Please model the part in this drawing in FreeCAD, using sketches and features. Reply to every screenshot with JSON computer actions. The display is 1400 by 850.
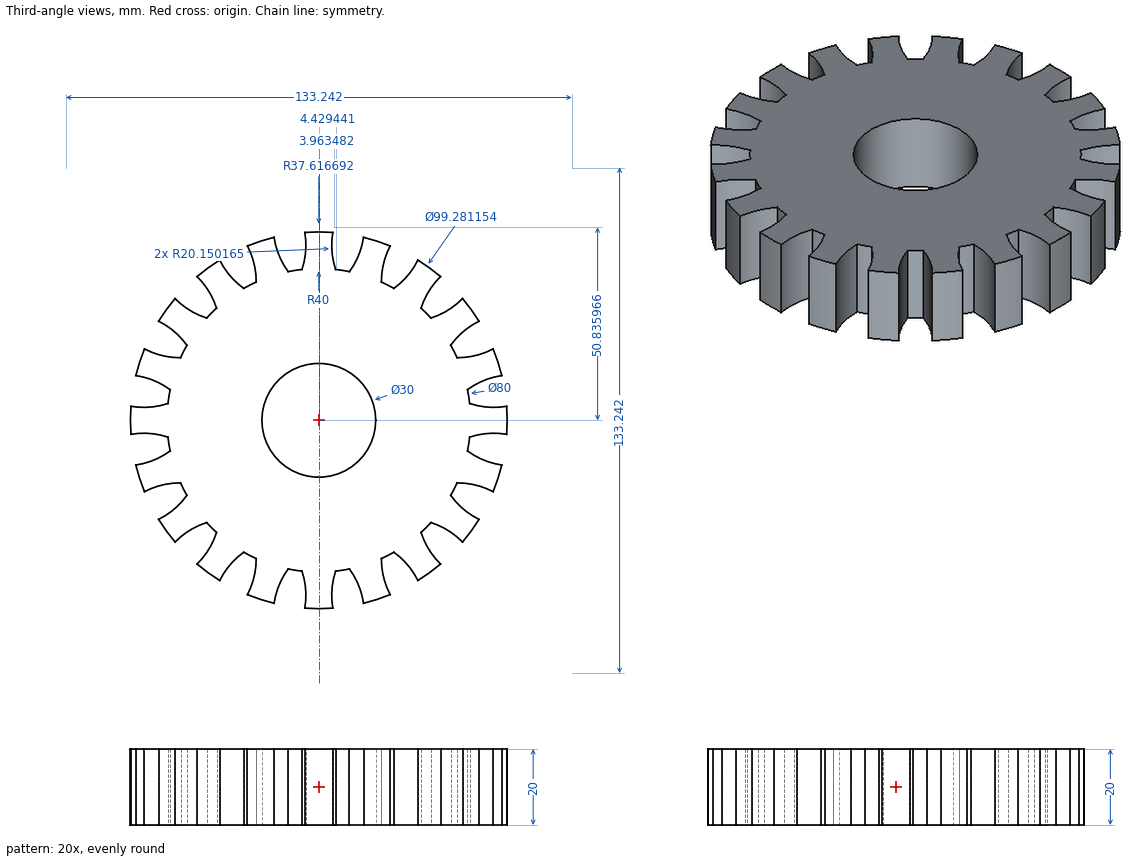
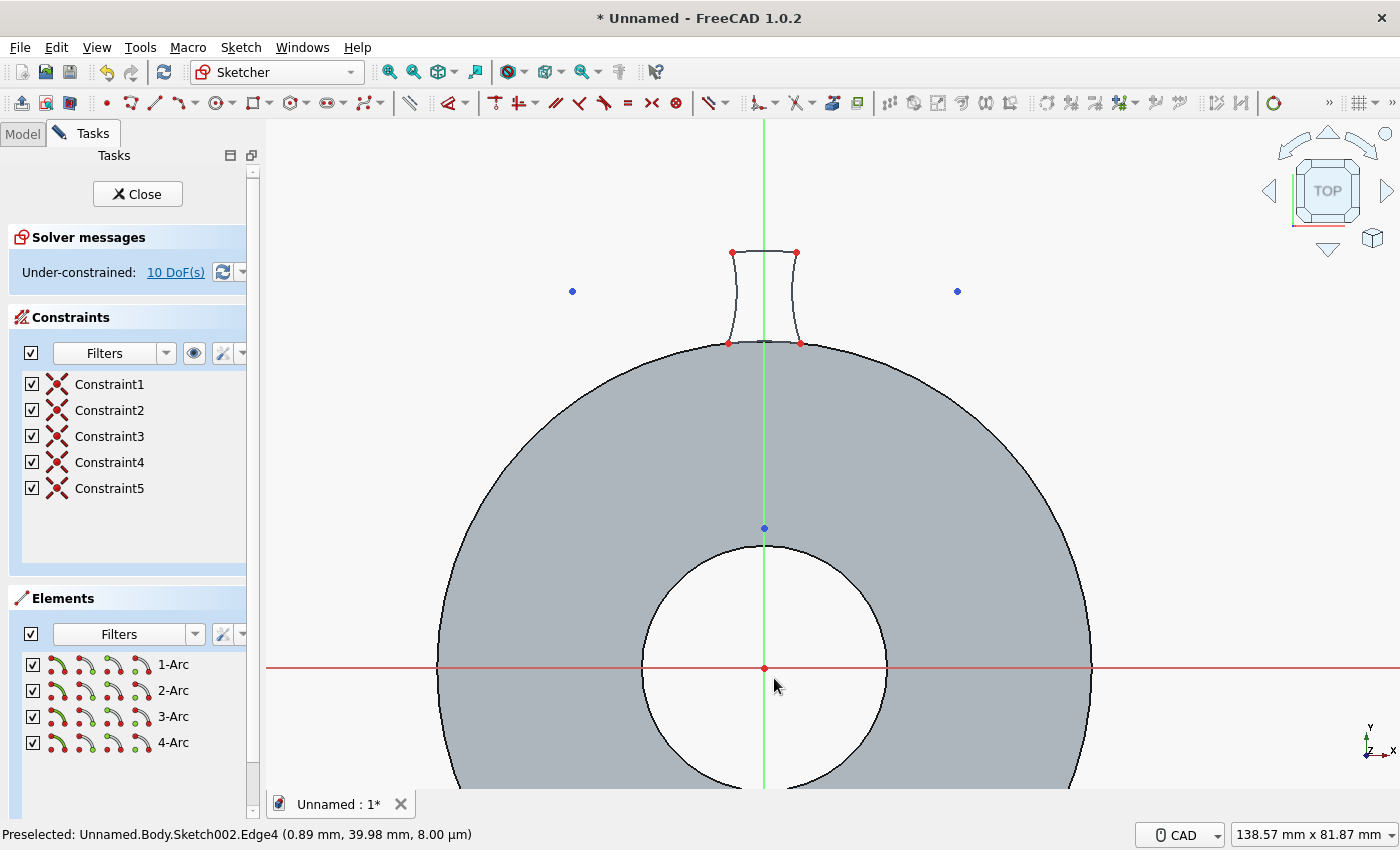
{"action": "left_click", "coordinate": [793, 280]}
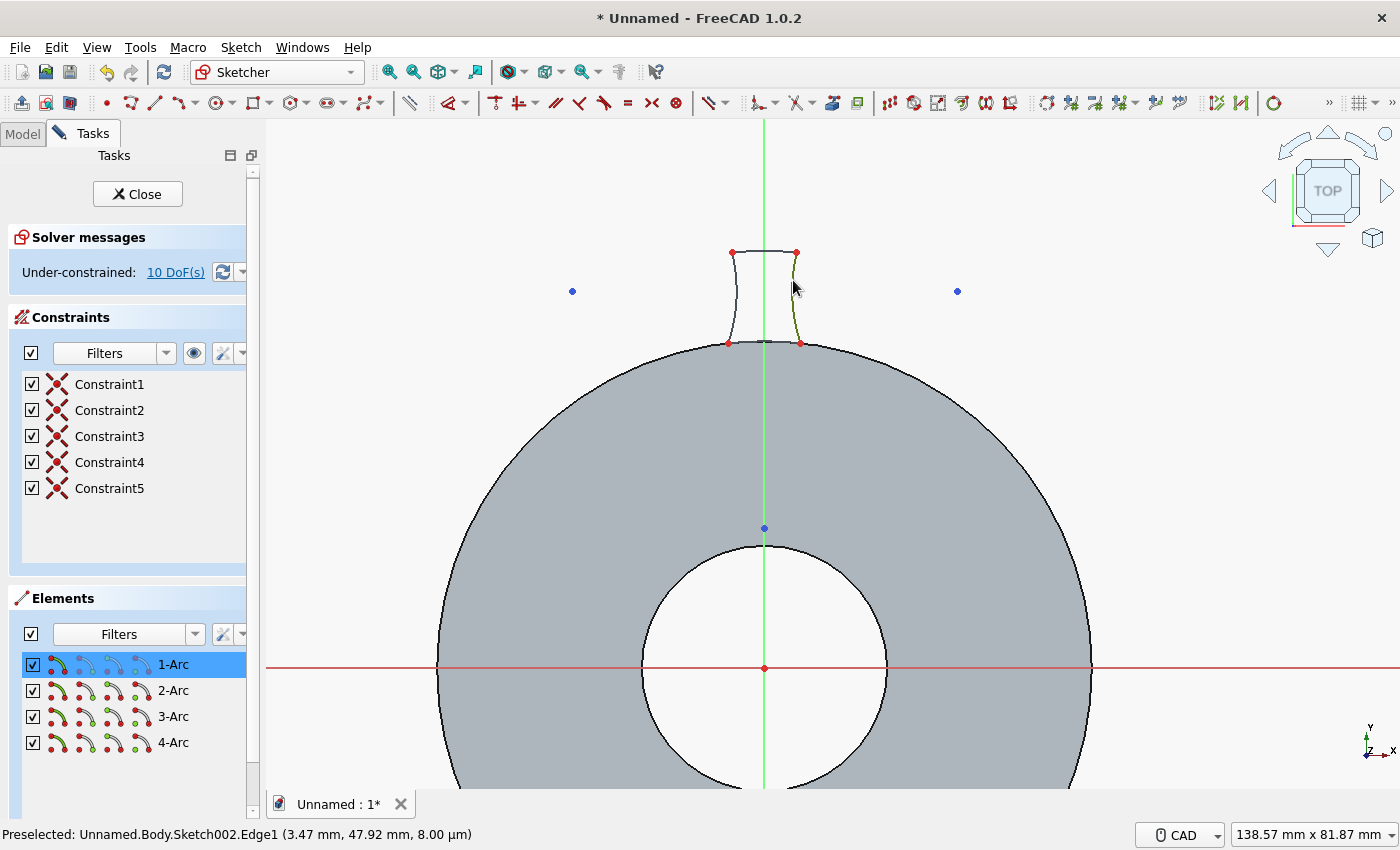
{"action": "left_click", "coordinate": [735, 317]}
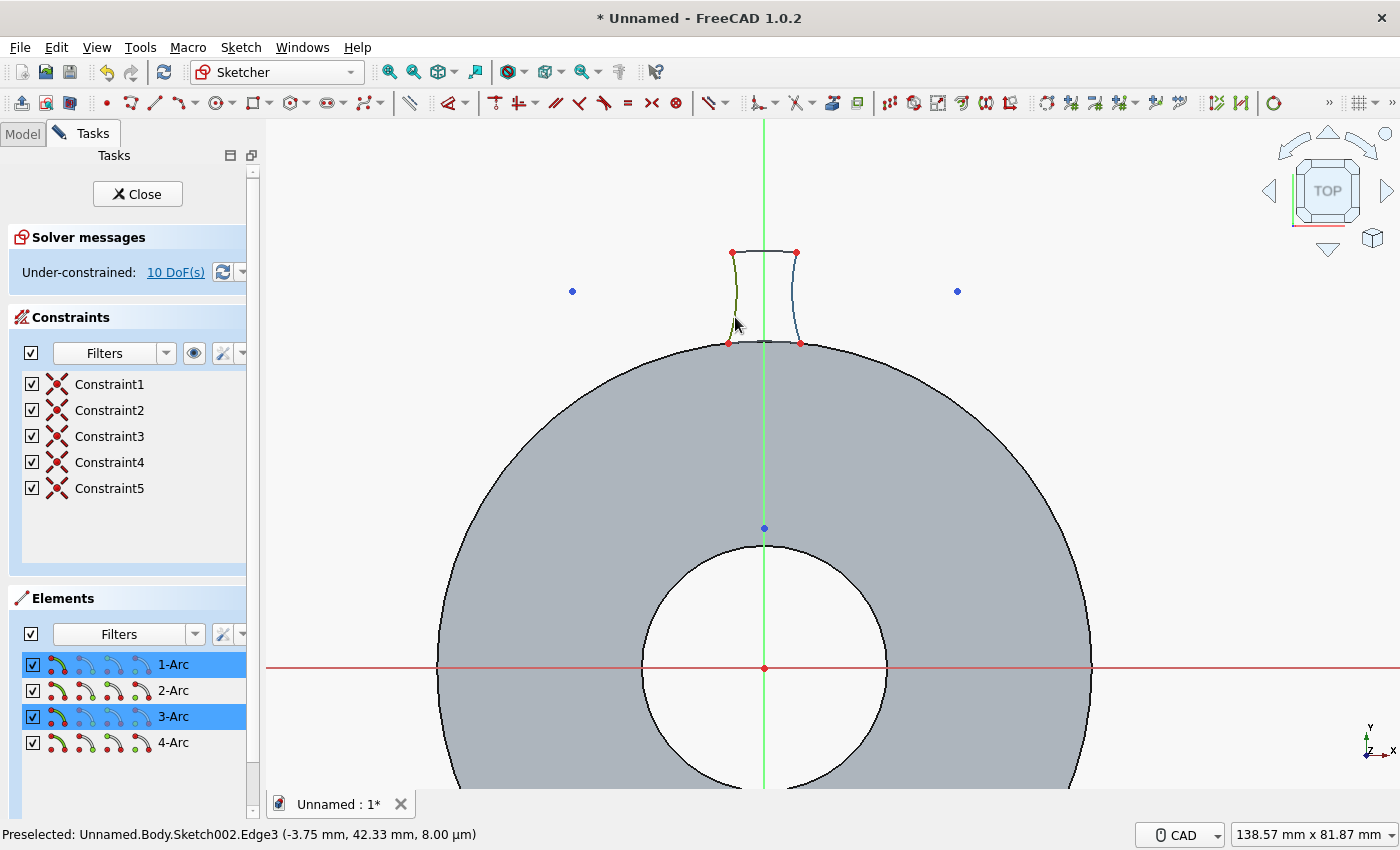
{"action": "left_click", "coordinate": [628, 104]}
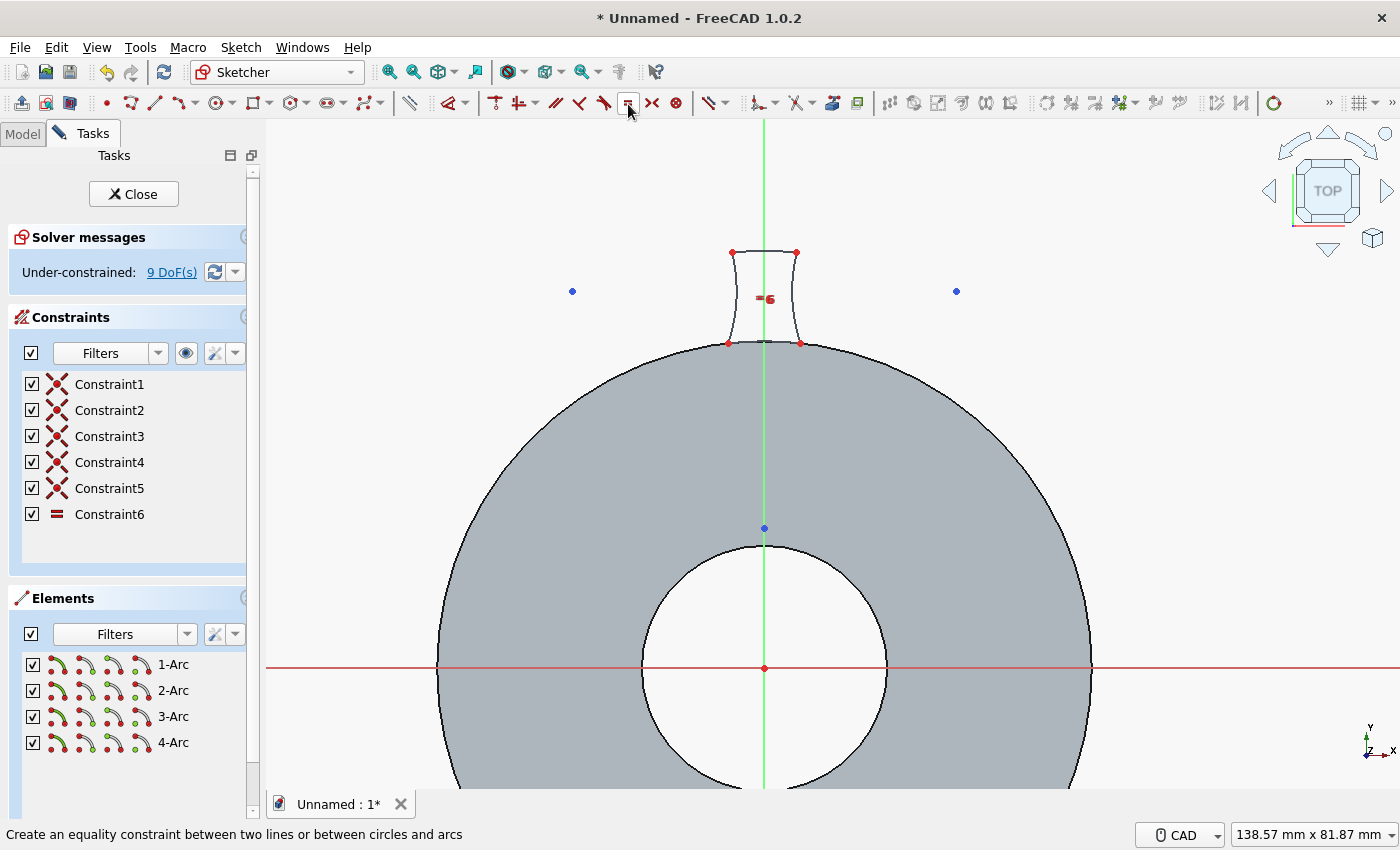
{"action": "left_click", "coordinate": [764, 529]}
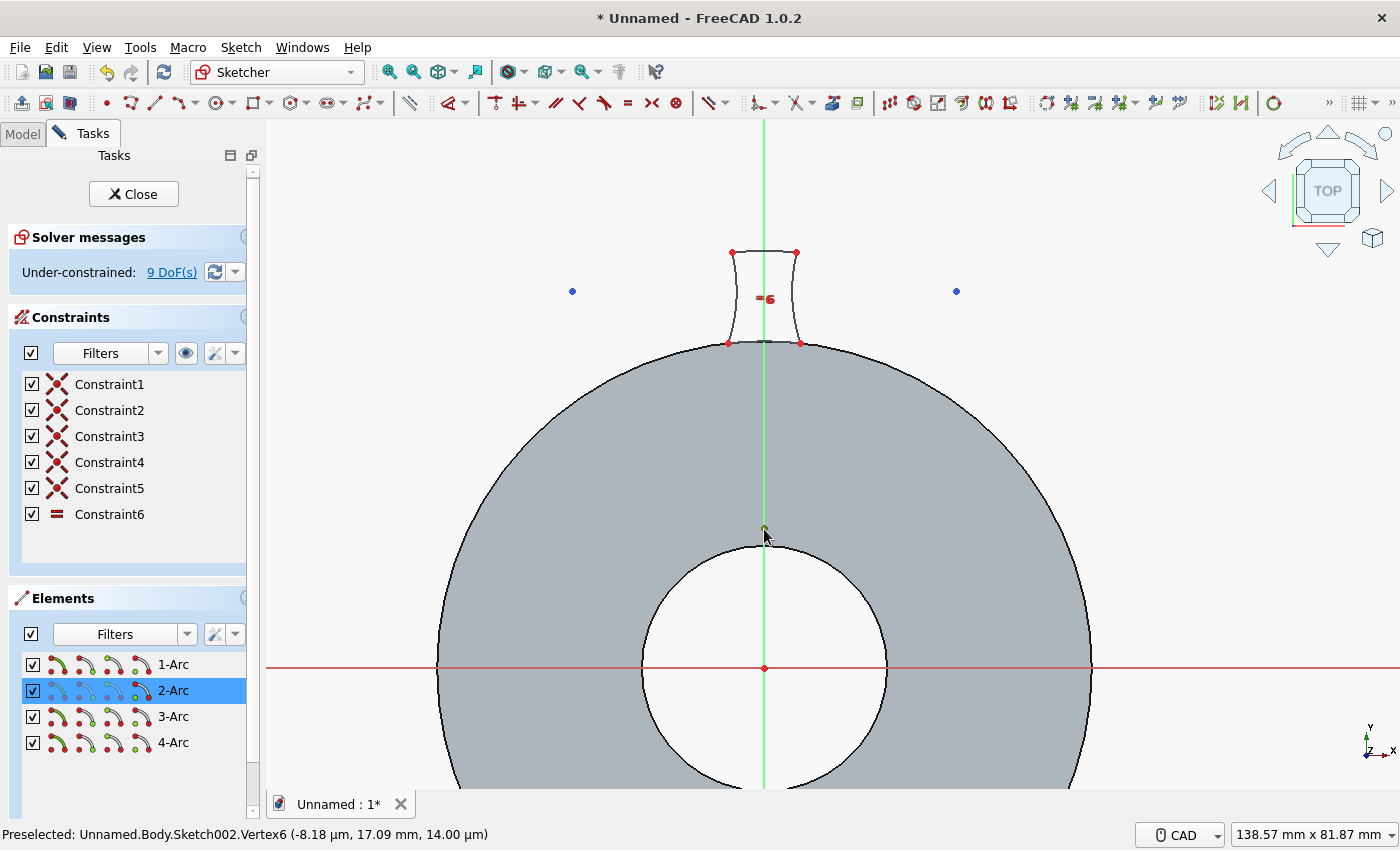
{"action": "left_click", "coordinate": [764, 717]}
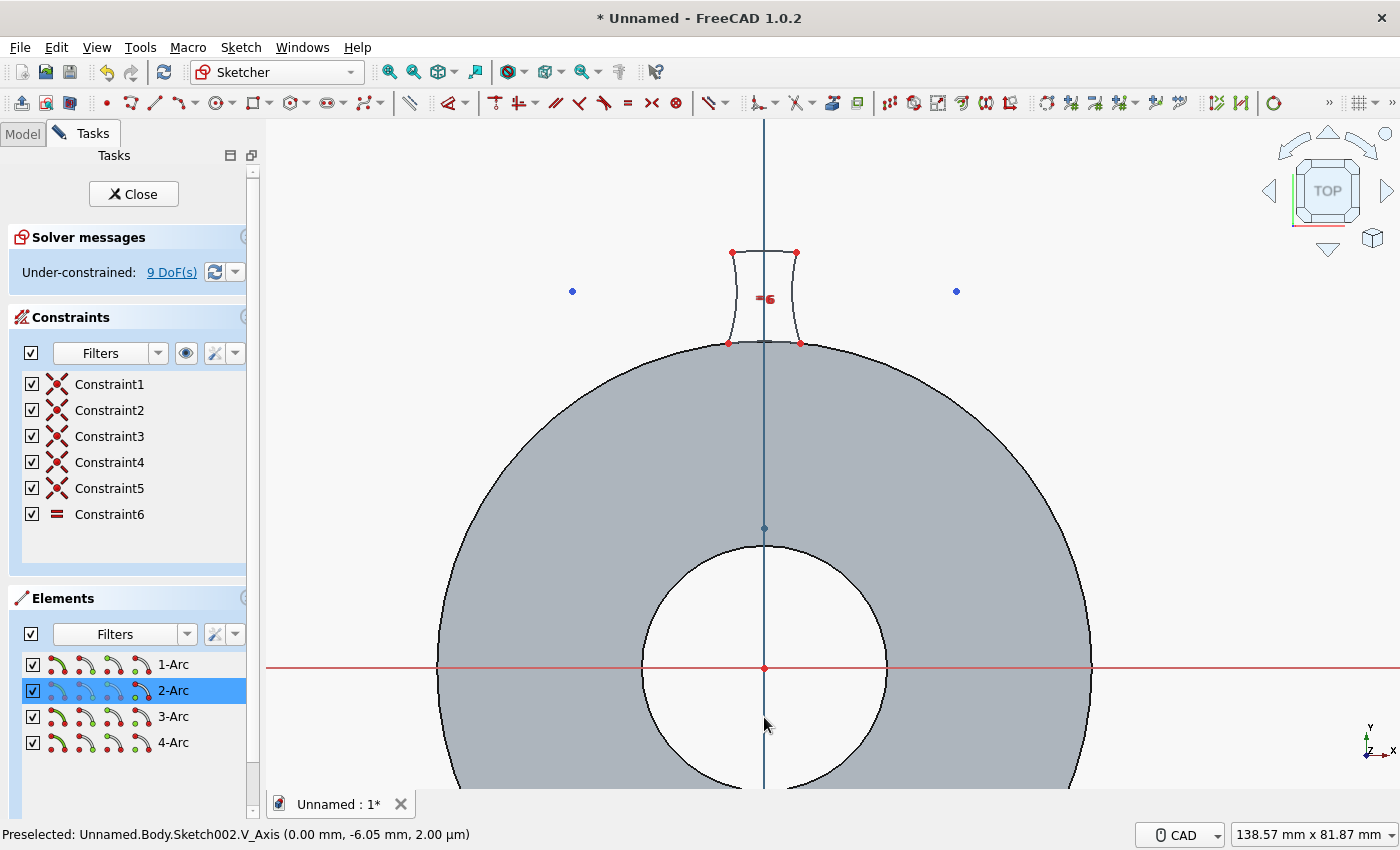
{"action": "left_click", "coordinate": [496, 104]}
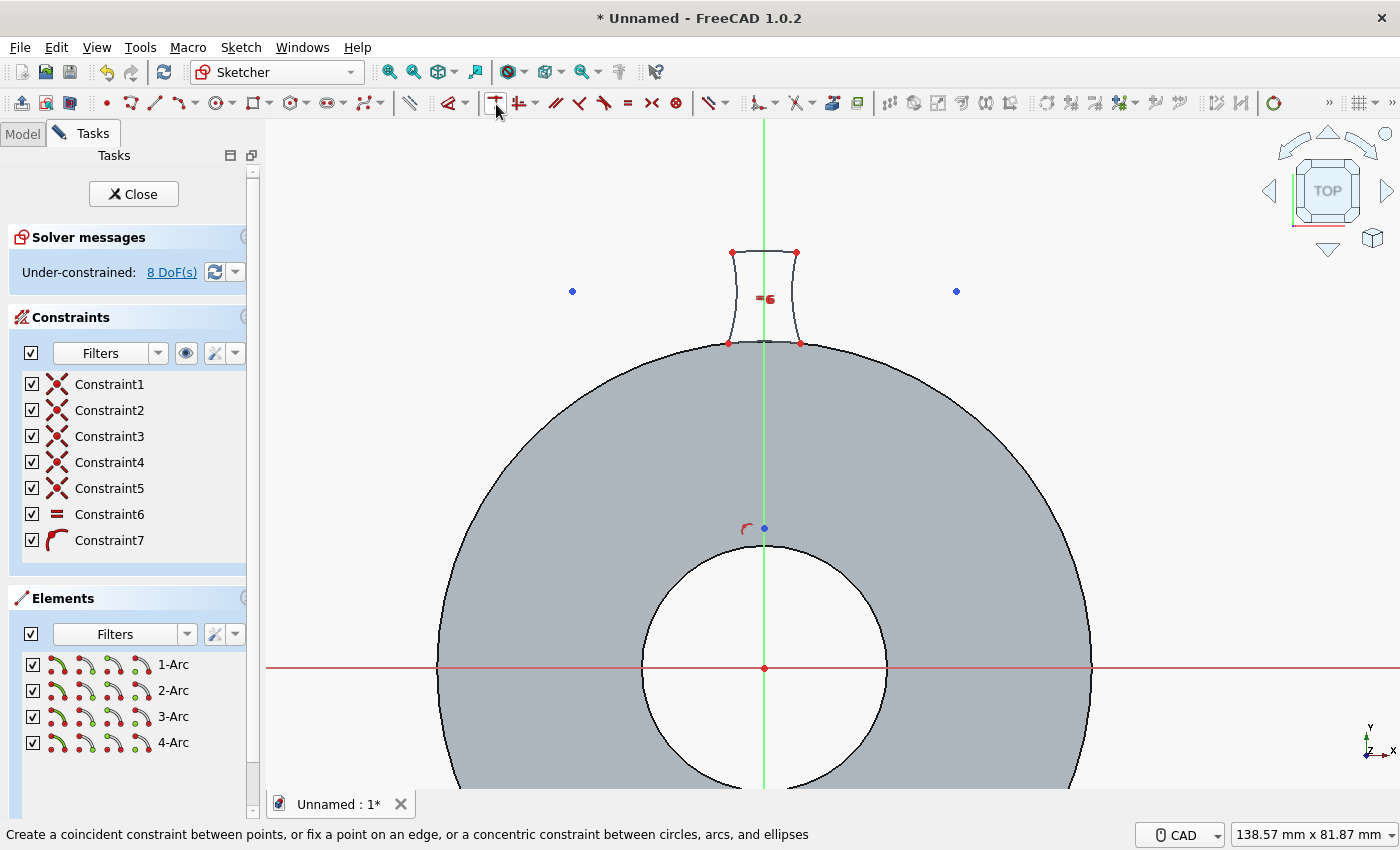
{"action": "left_click", "coordinate": [956, 291]}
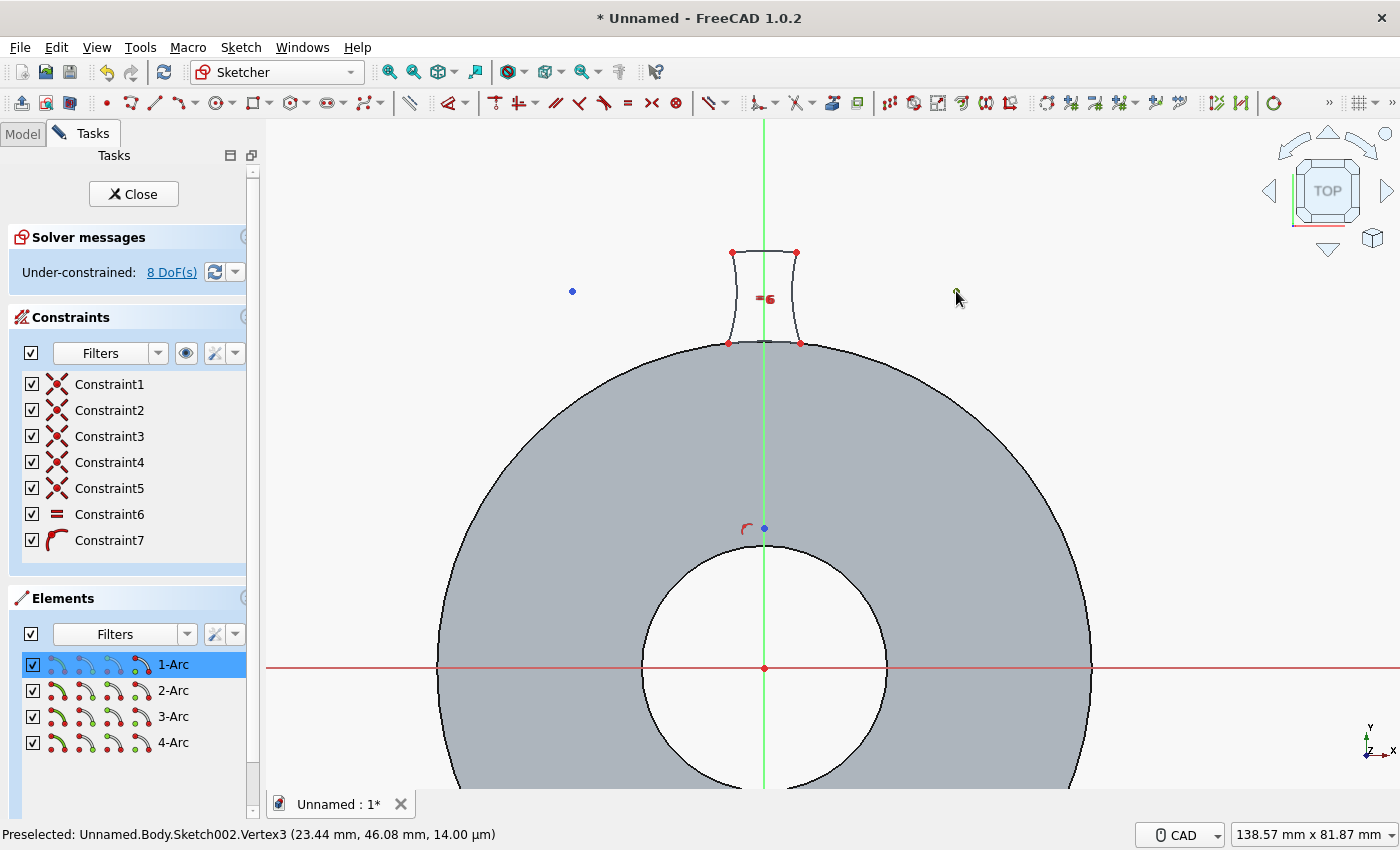
{"action": "left_click", "coordinate": [573, 291]}